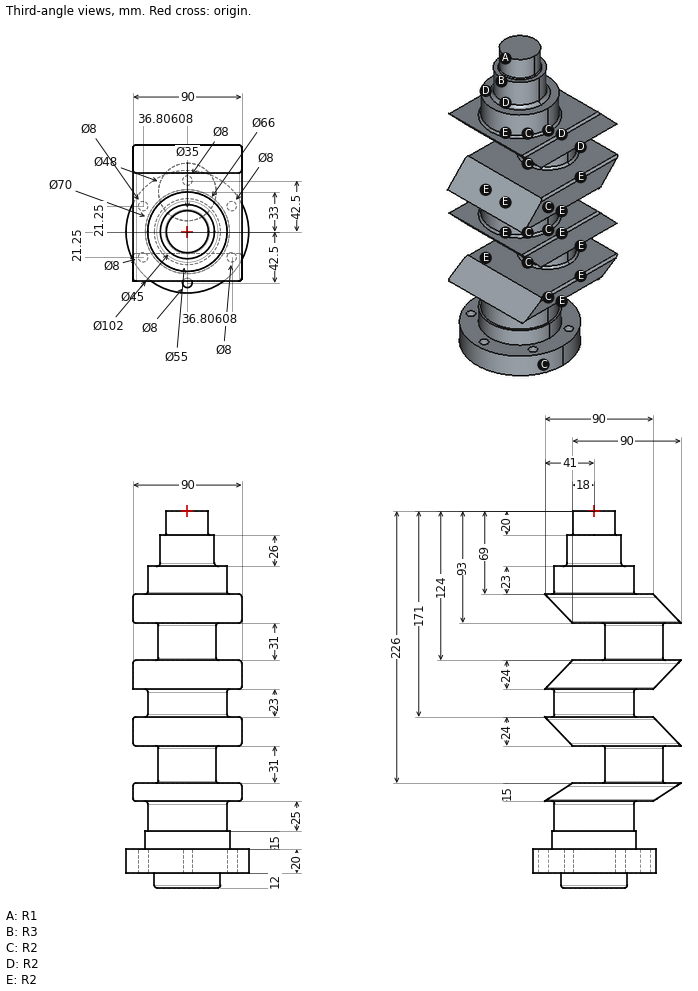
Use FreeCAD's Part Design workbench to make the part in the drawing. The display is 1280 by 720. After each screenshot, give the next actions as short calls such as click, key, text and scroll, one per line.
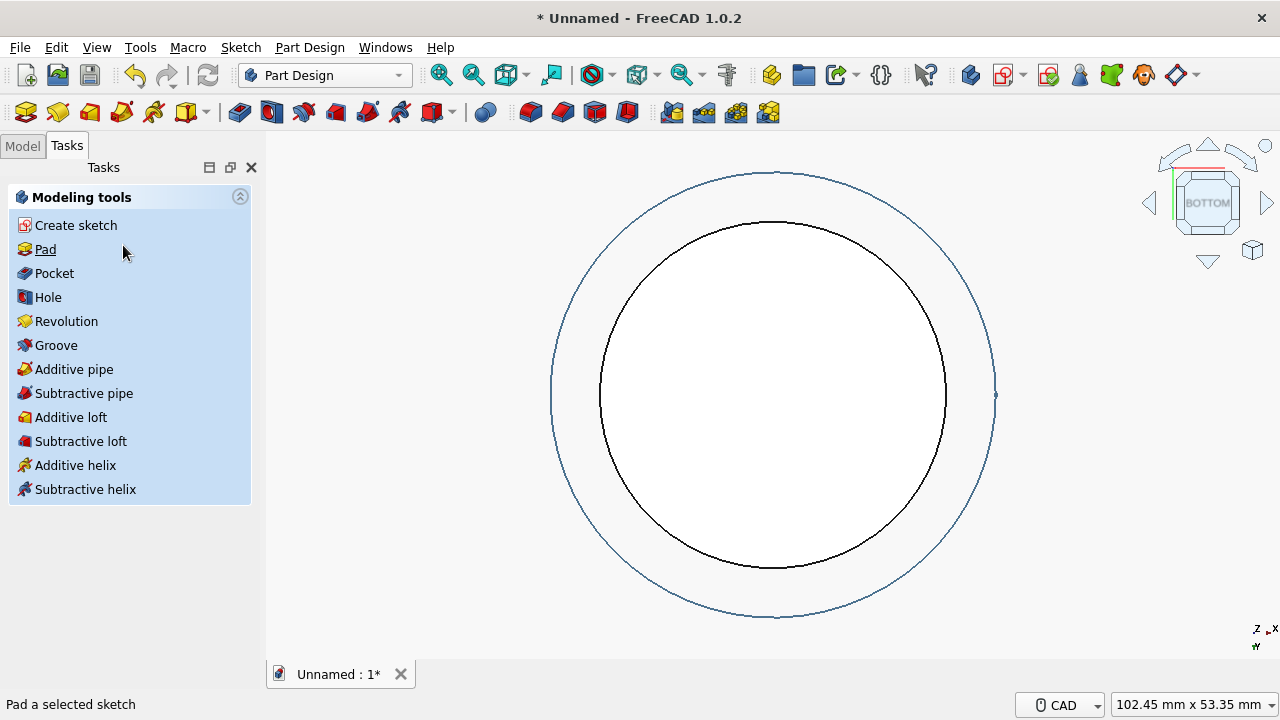
click(26, 112)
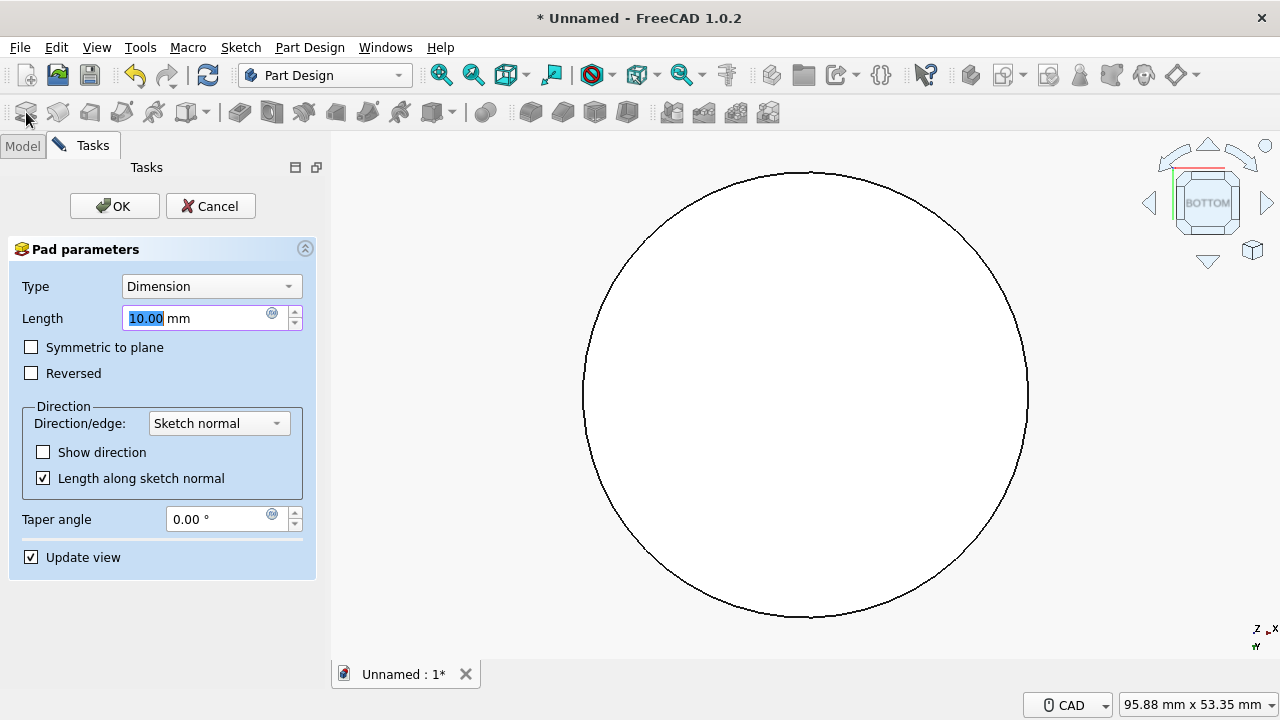
text(26)
key(Tab)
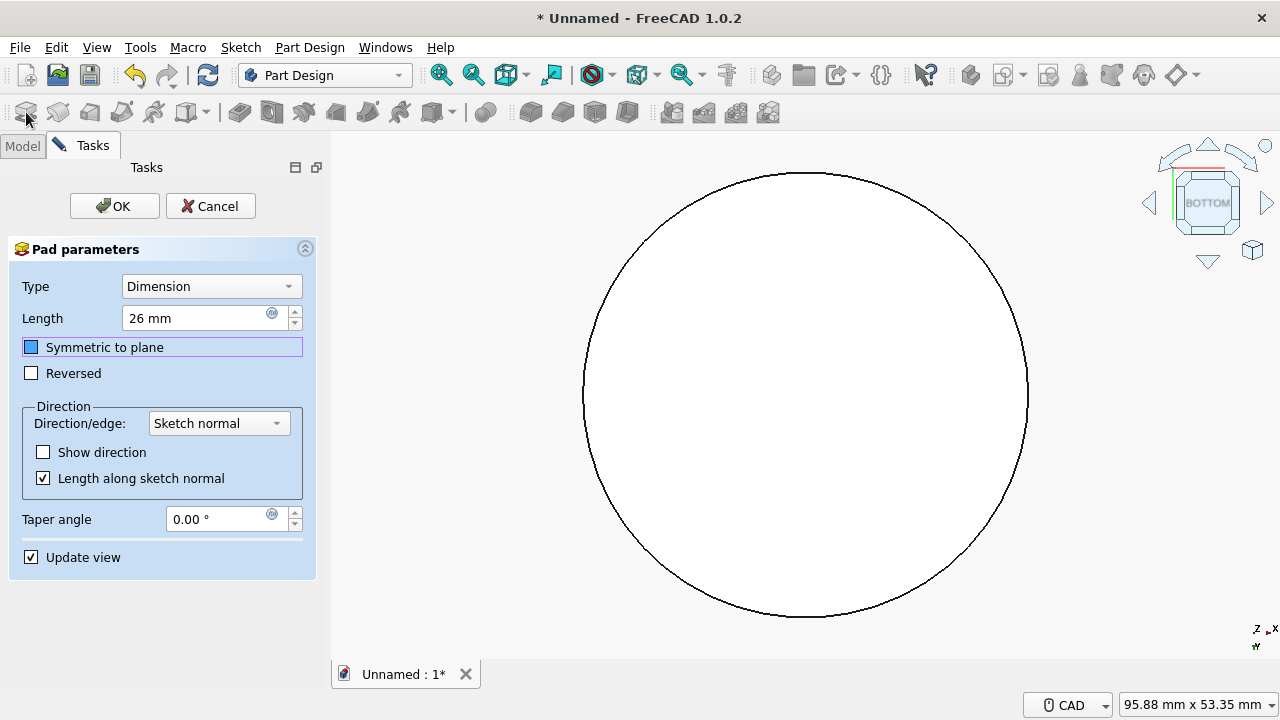
click(115, 206)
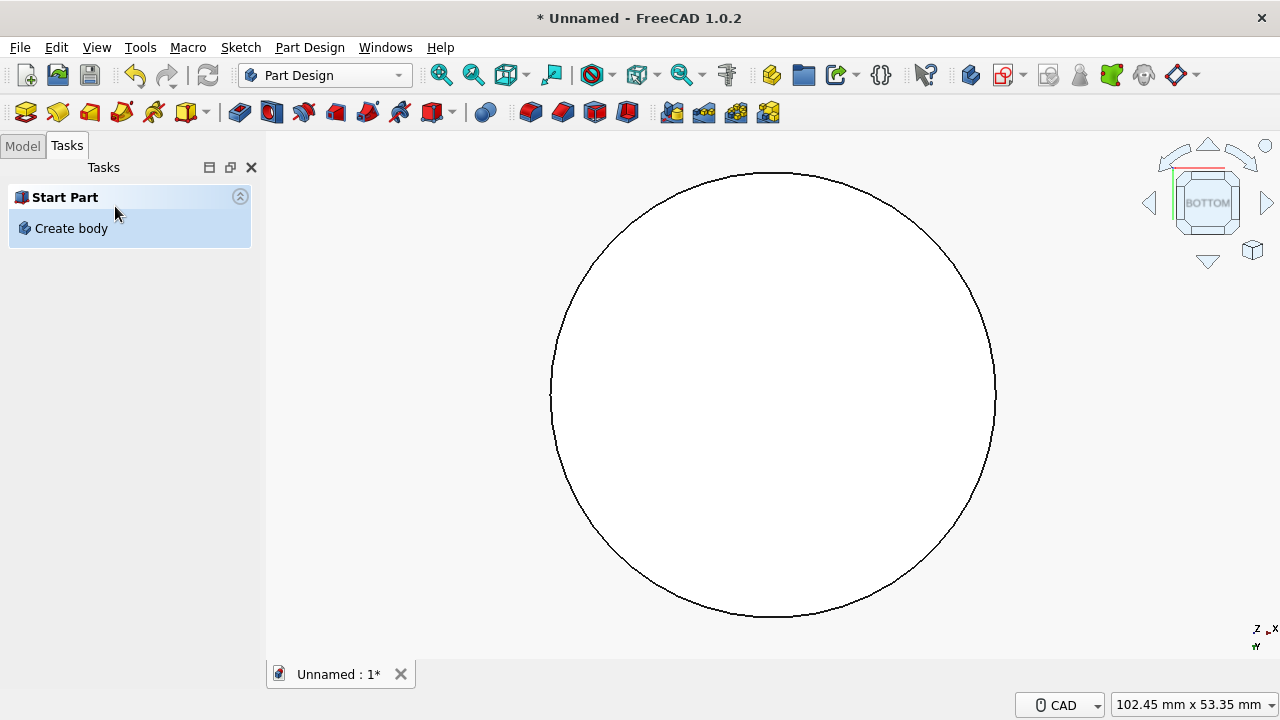
click(773, 394)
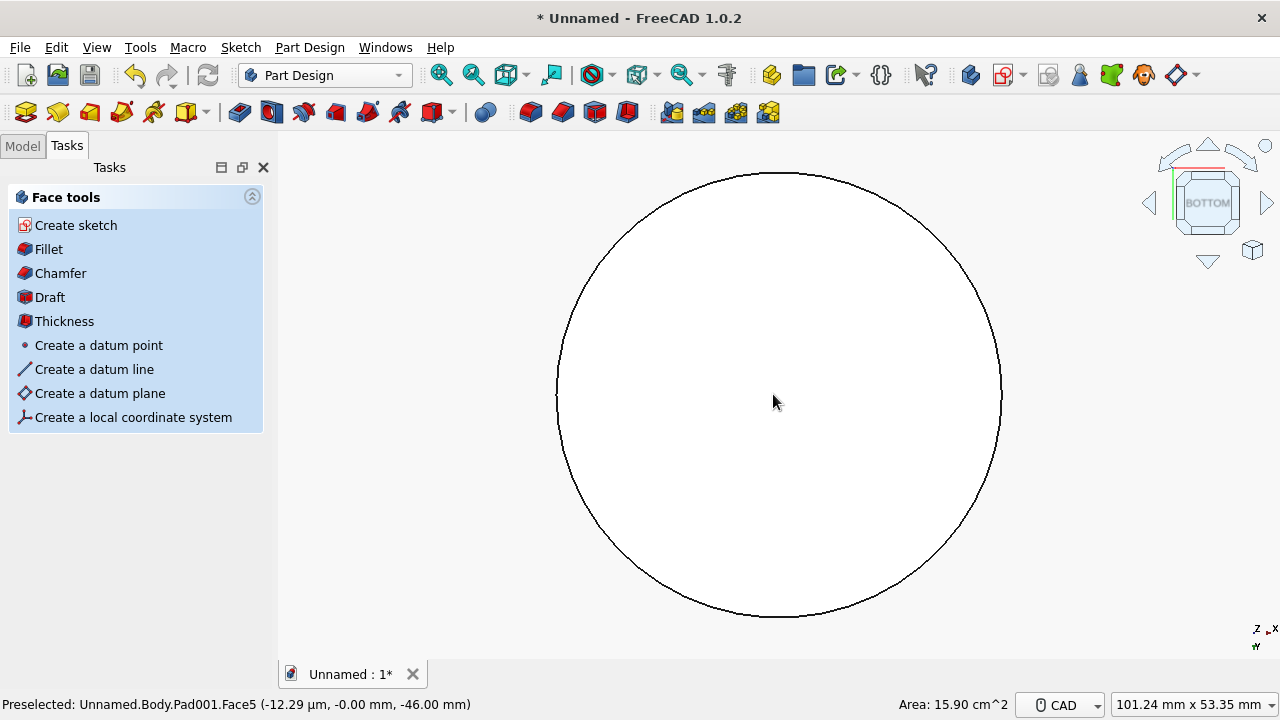
click(1004, 76)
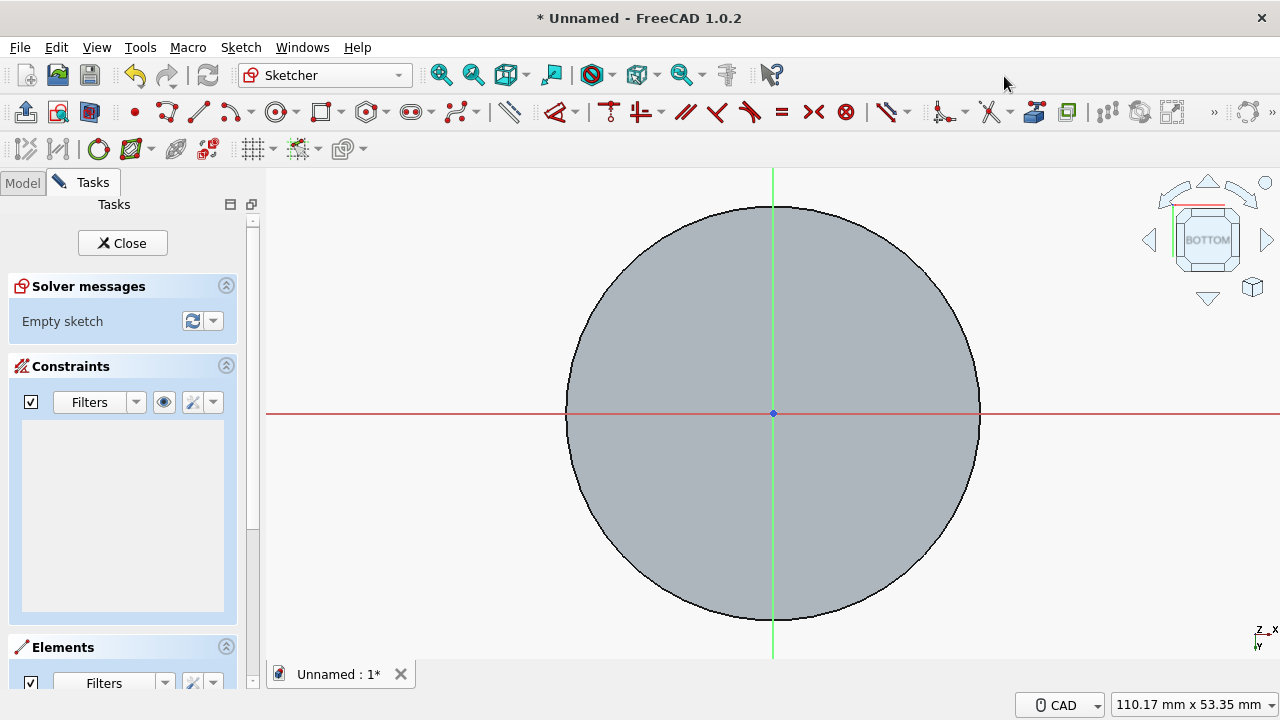
scroll(621, 413, down, 3)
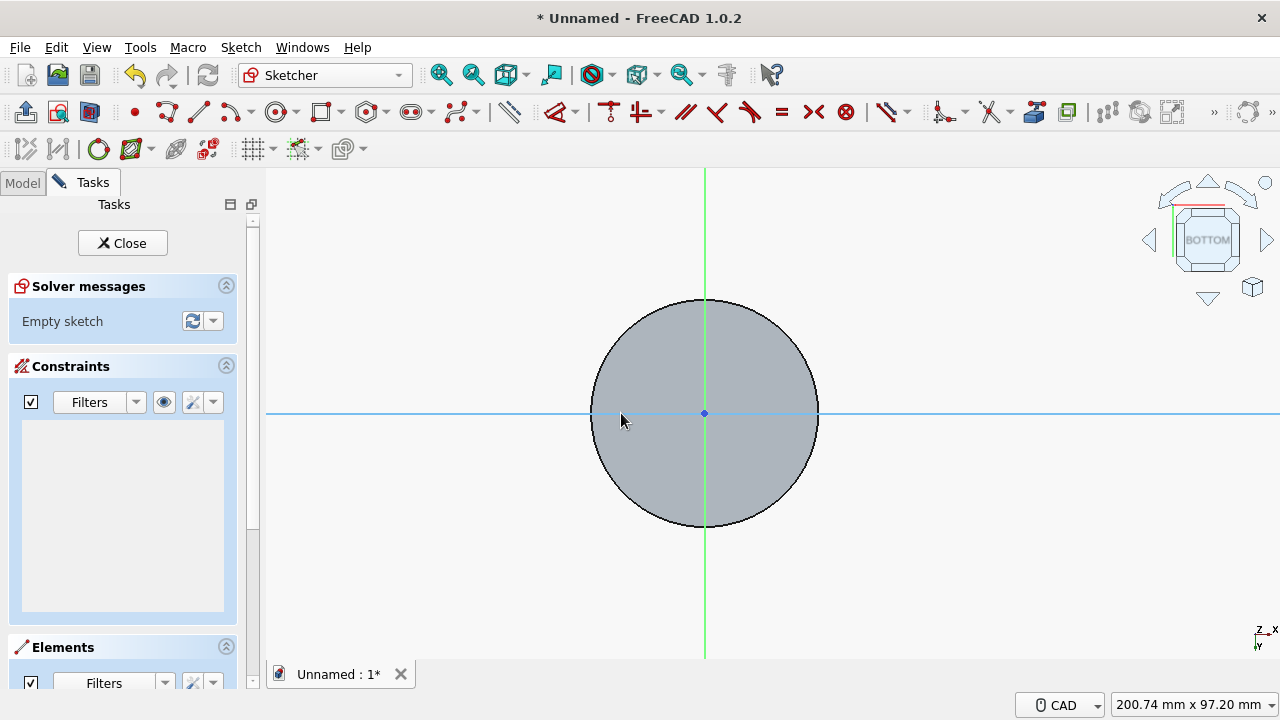
click(276, 112)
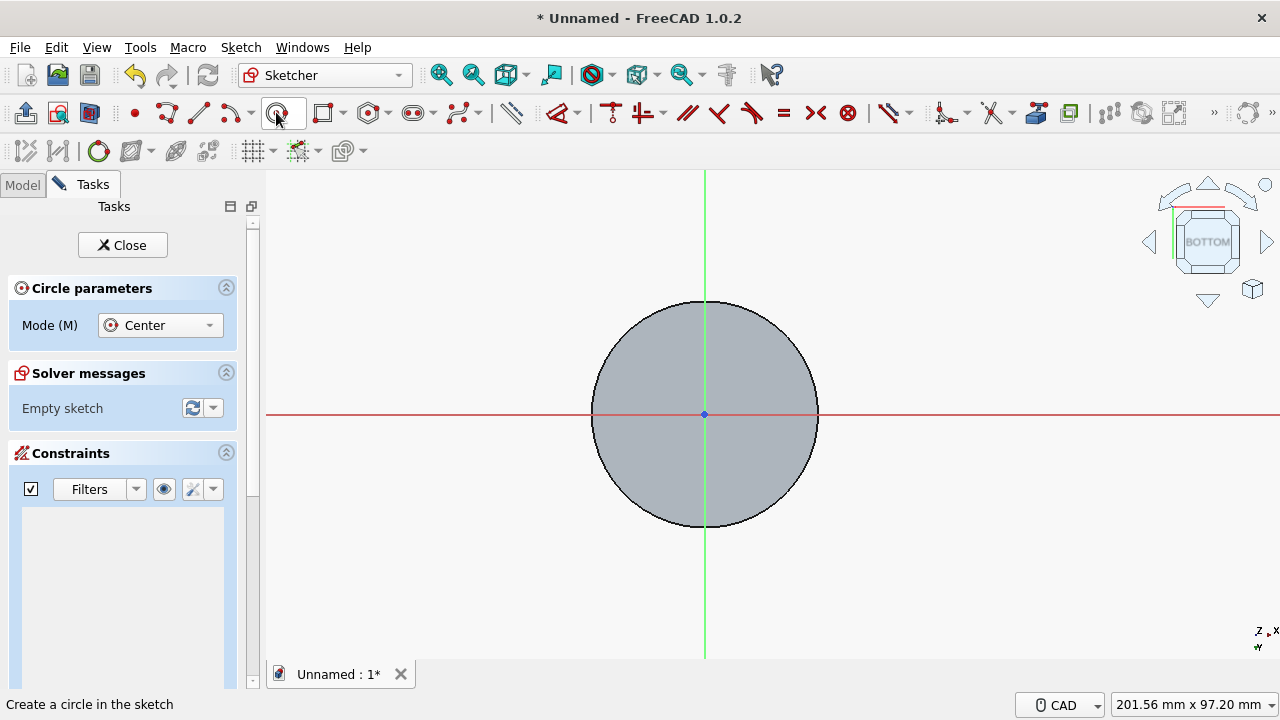
click(705, 415)
move(822, 297)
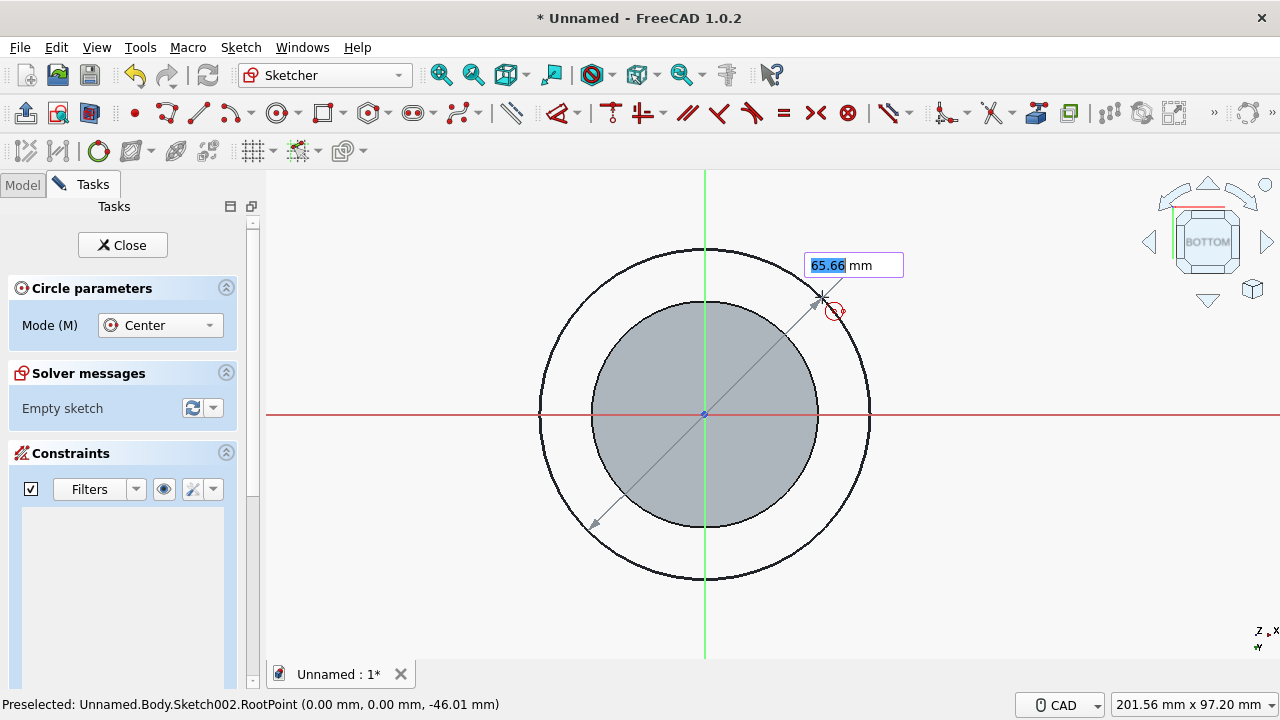
text(66)
key(Return)
key(Escape)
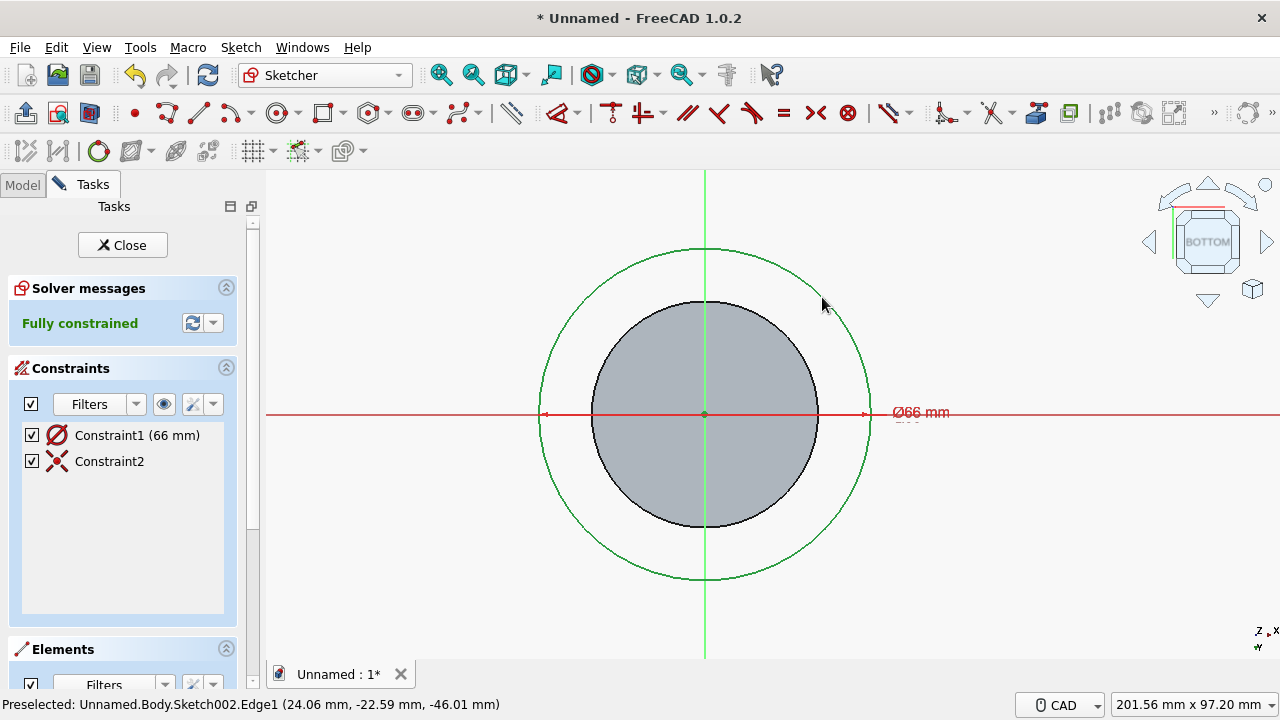
click(123, 245)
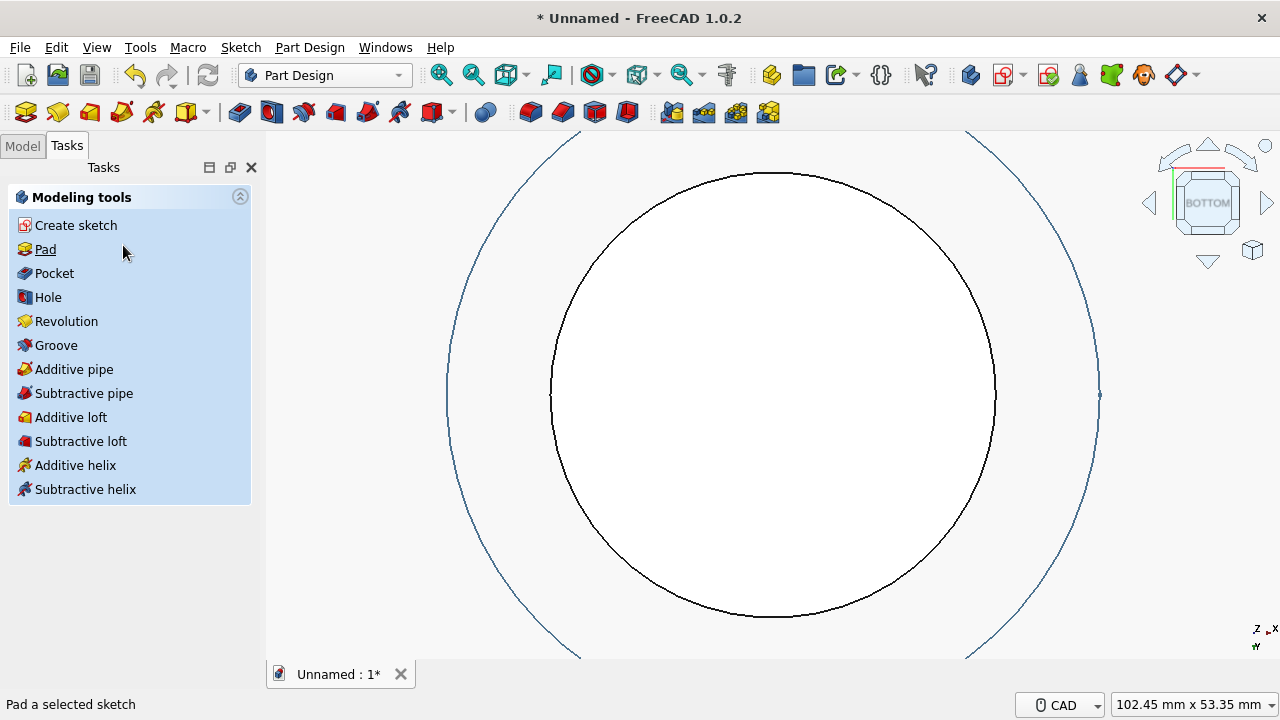
click(26, 112)